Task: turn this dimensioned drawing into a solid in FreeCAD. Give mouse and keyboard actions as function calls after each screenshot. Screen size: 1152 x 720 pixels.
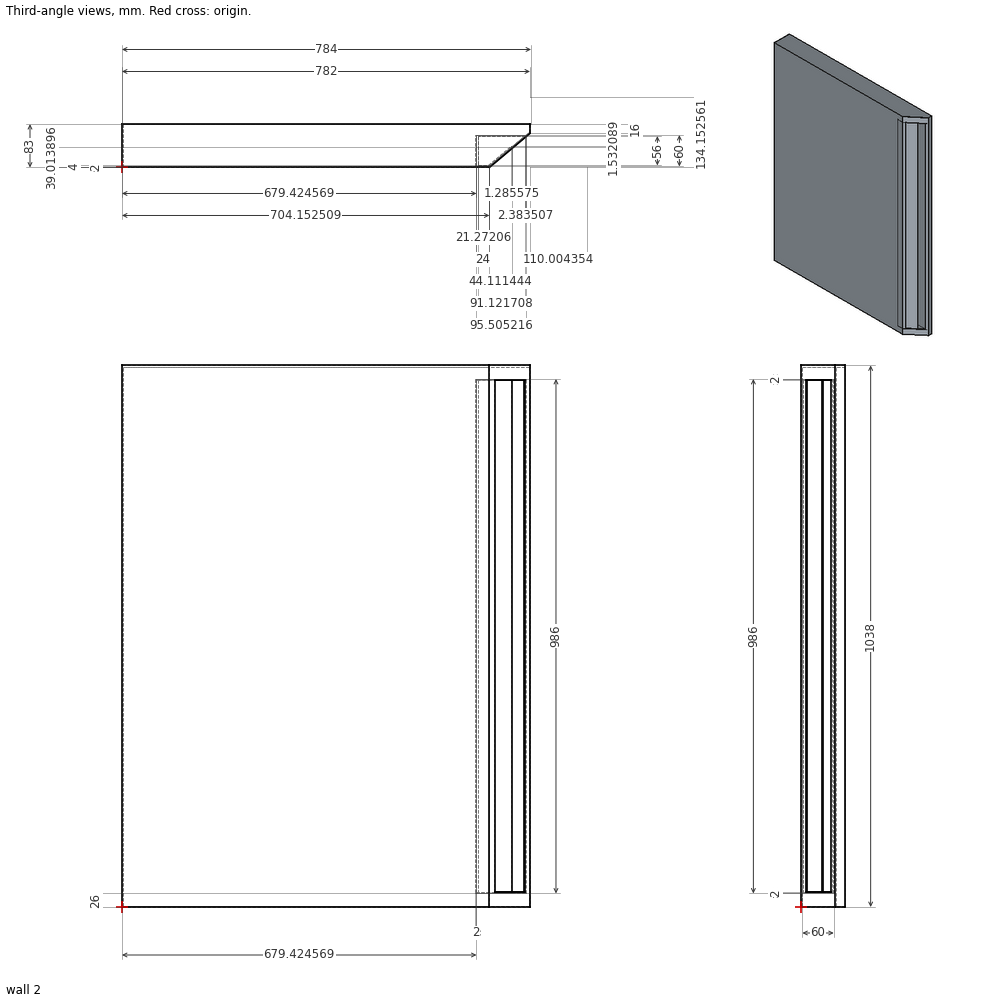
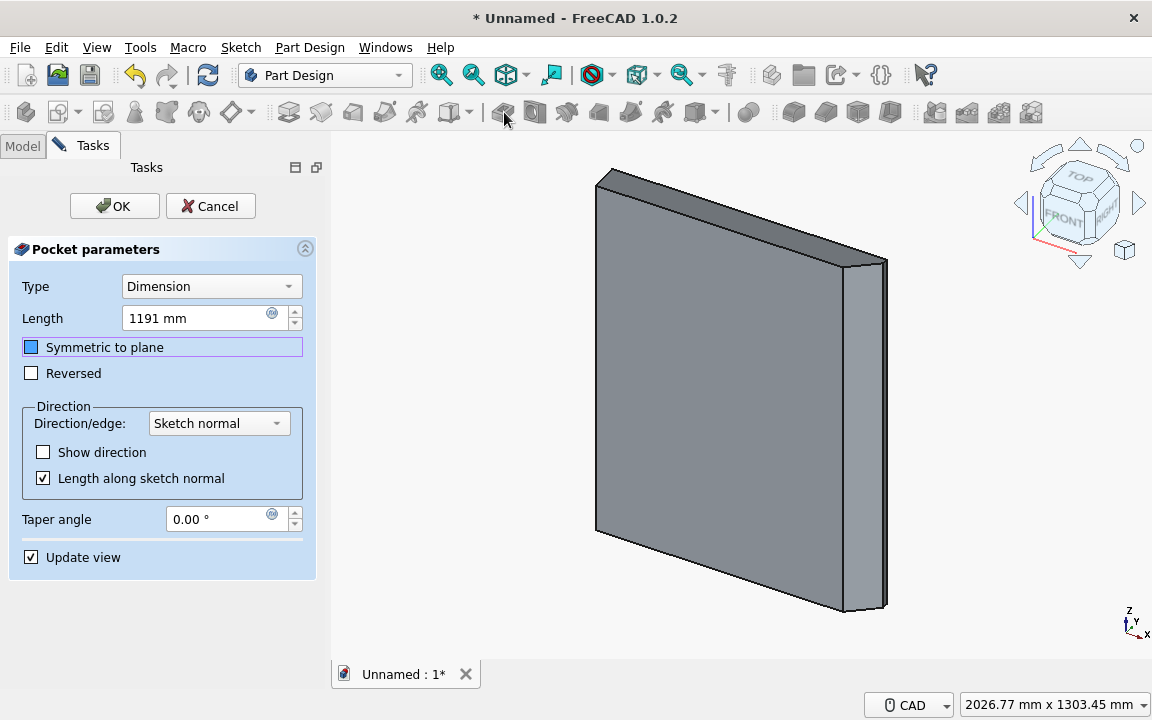
click(115, 206)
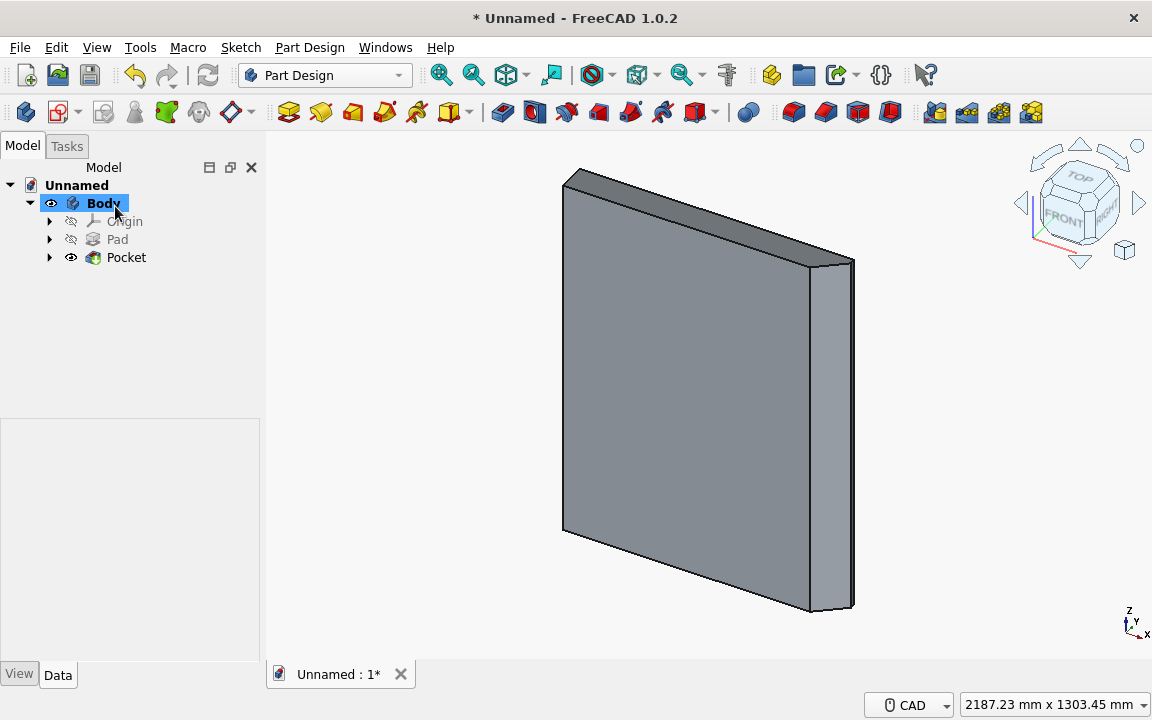
key(0)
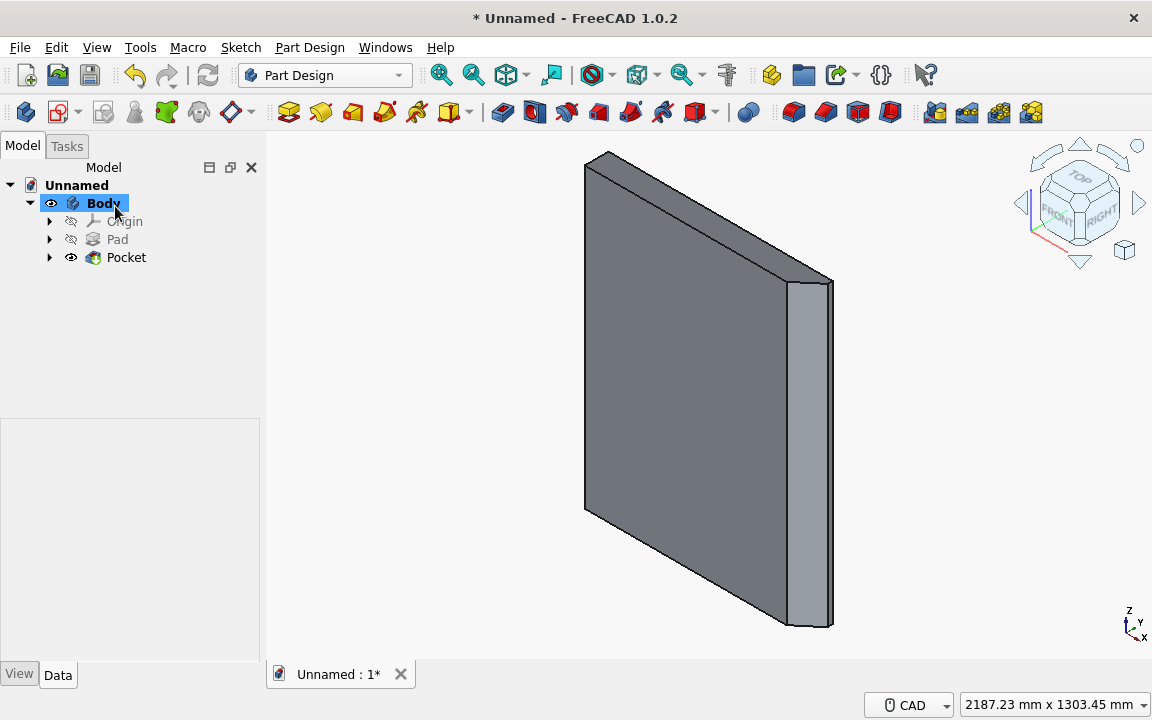
key(2)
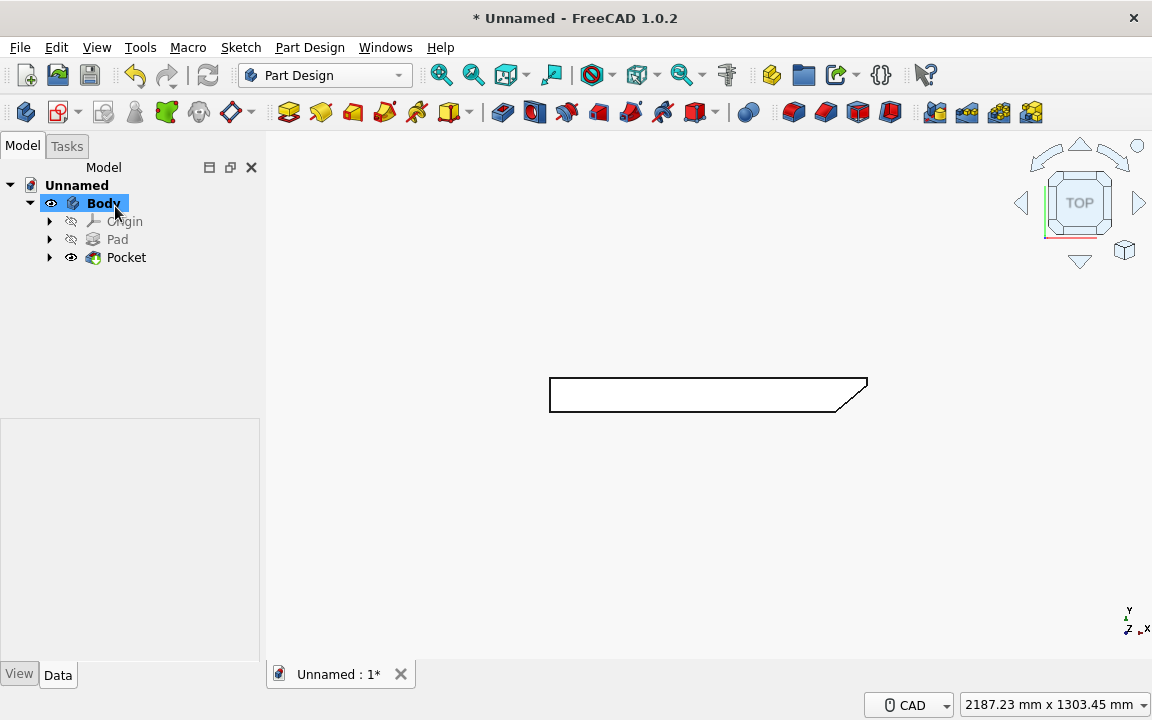
click(442, 76)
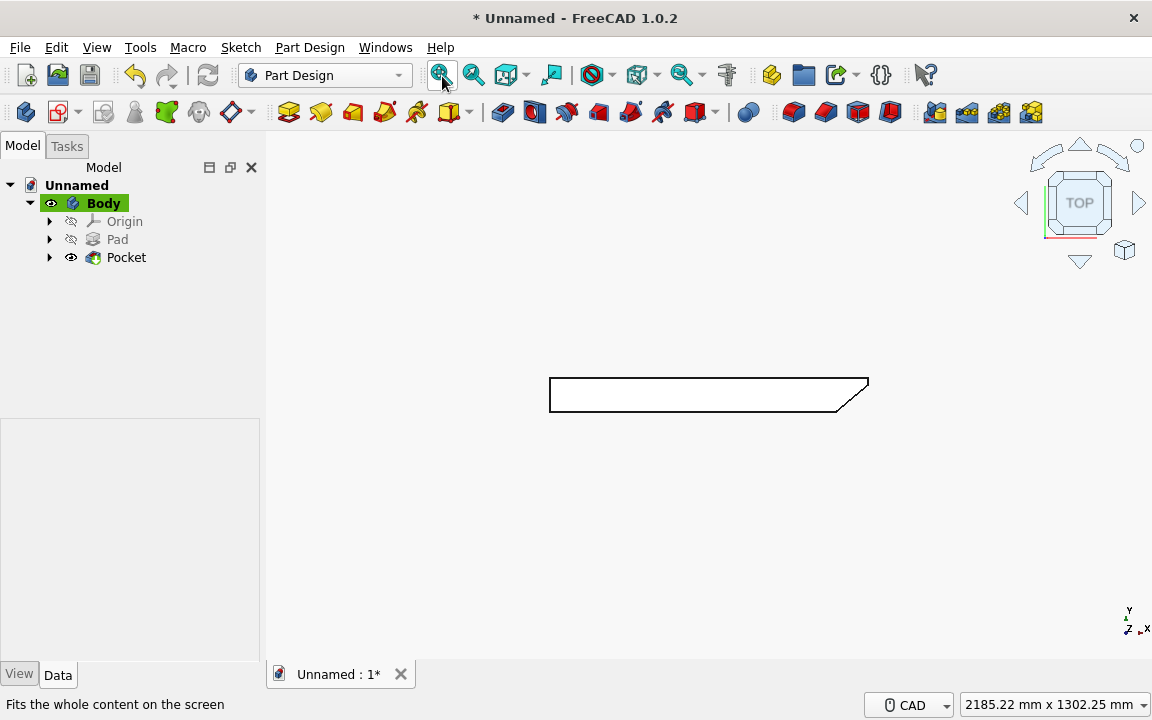
key(1)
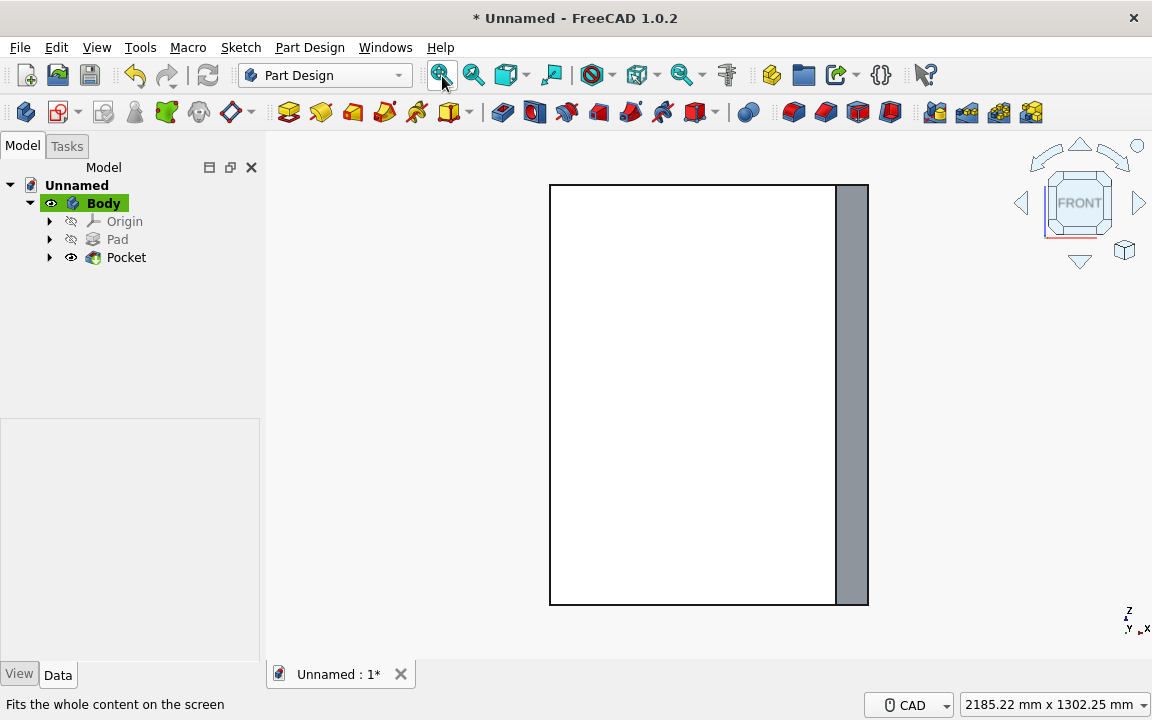
key(3)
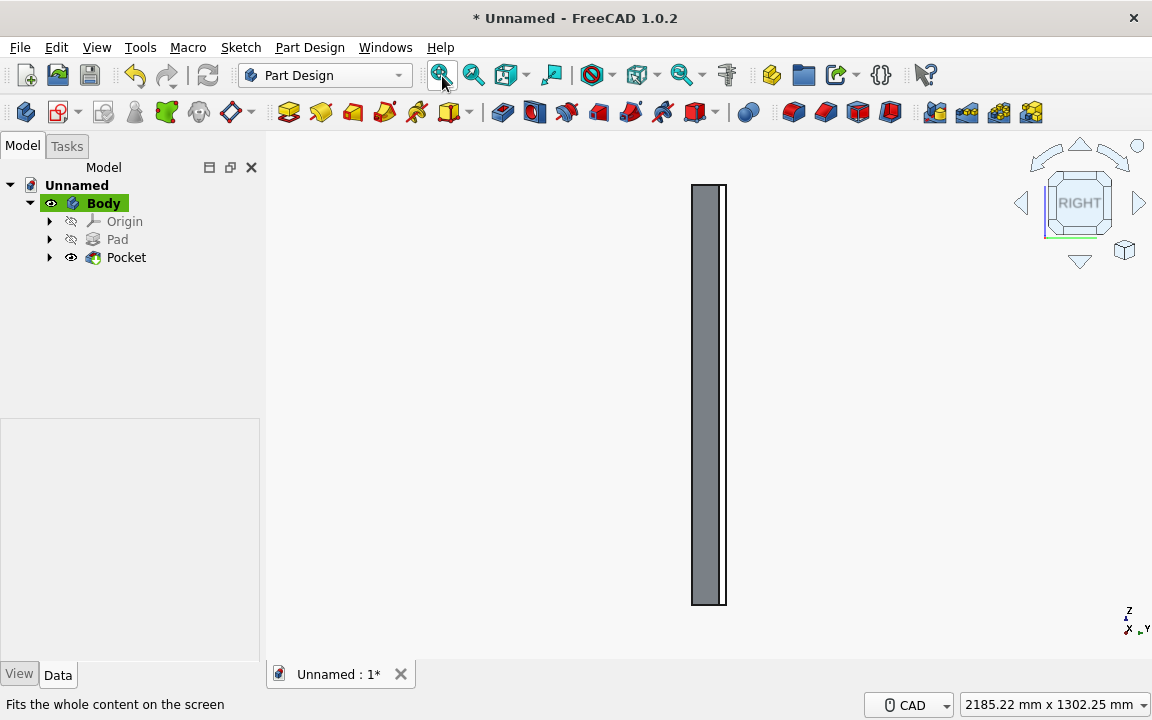
key(5)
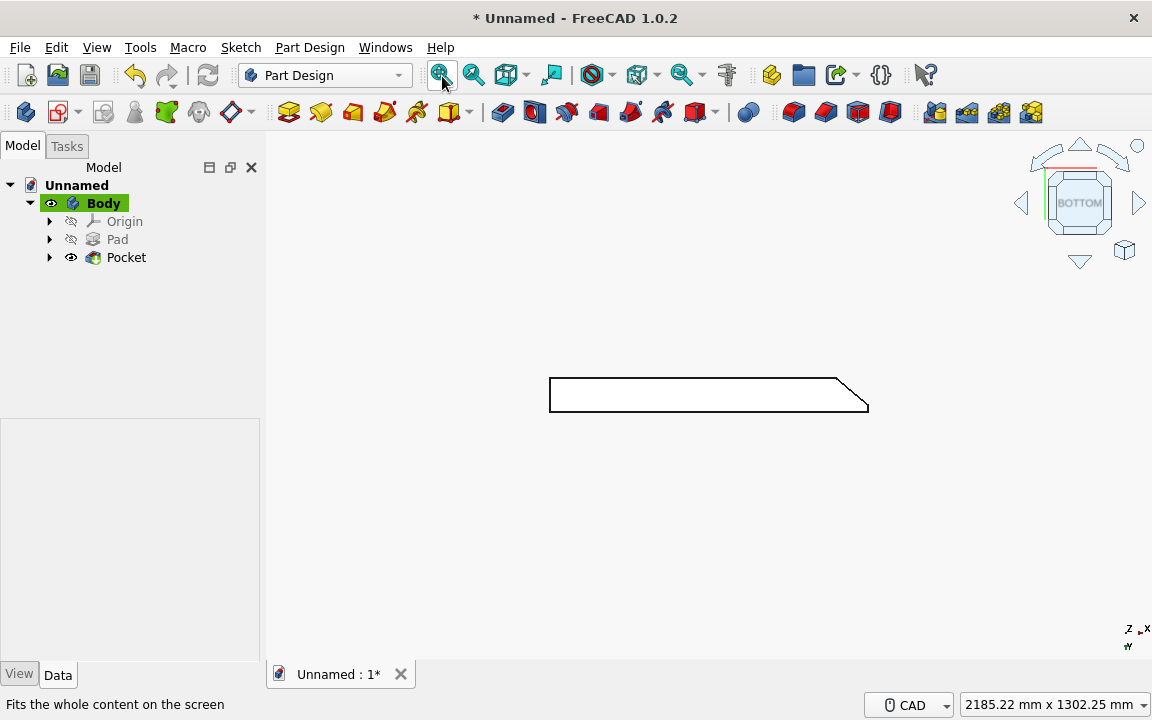
key(v)
key(f)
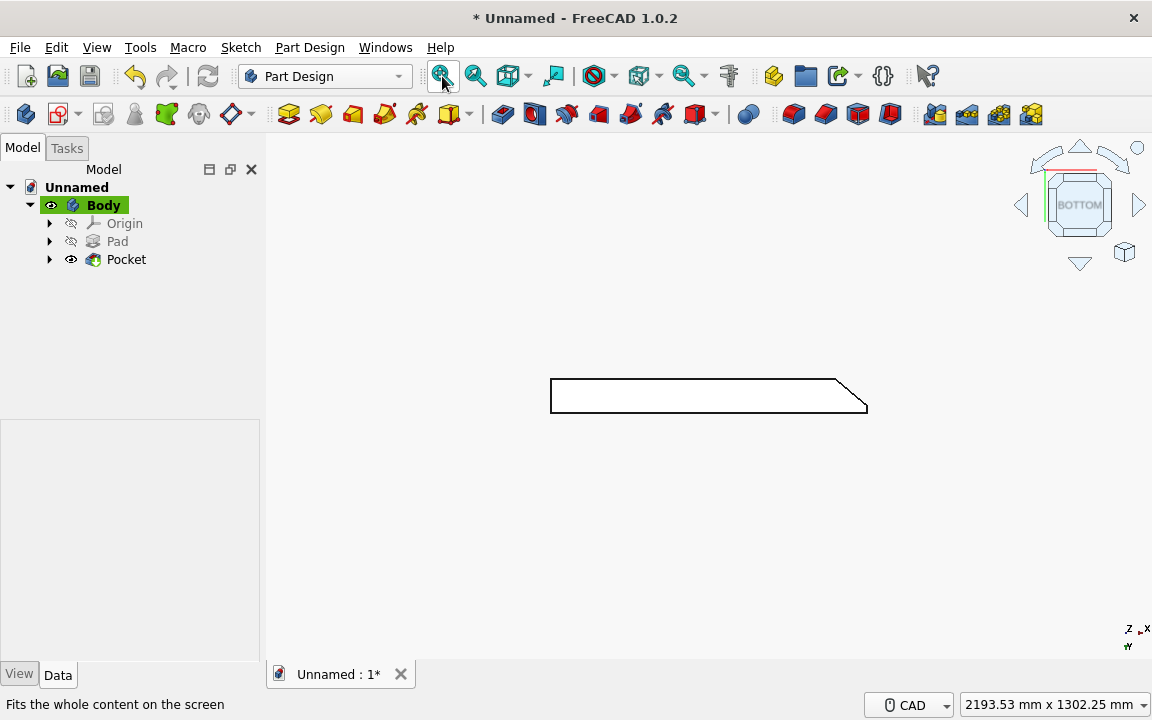
key(4)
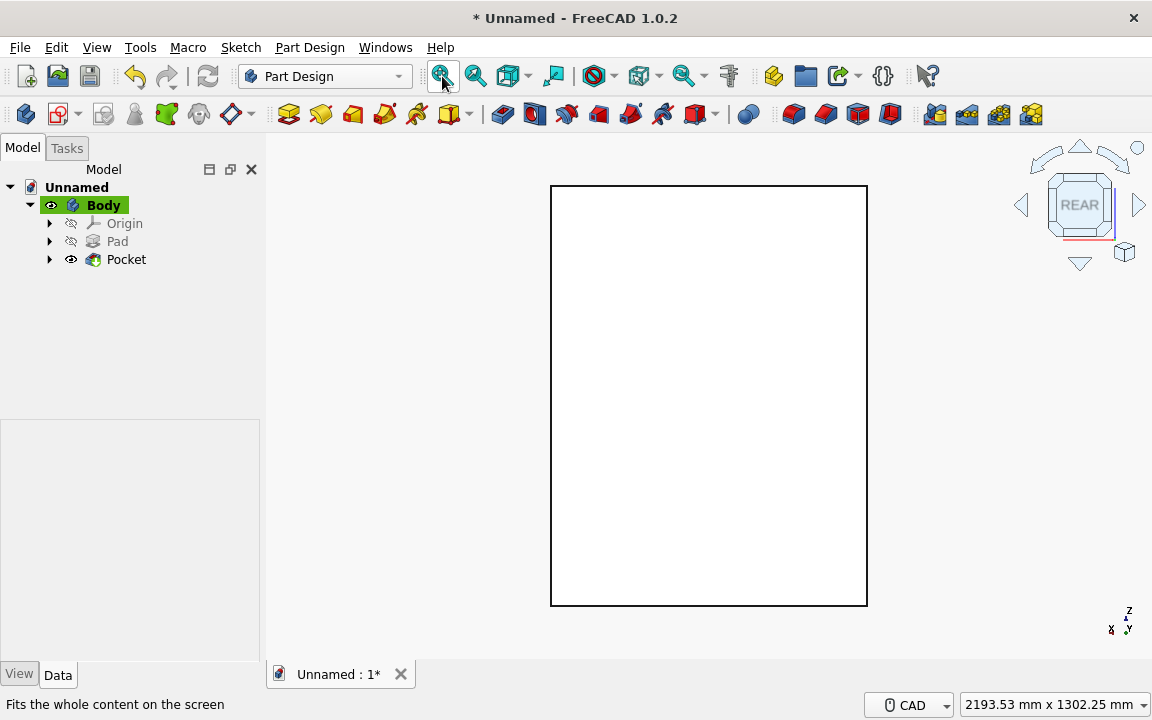
click(709, 395)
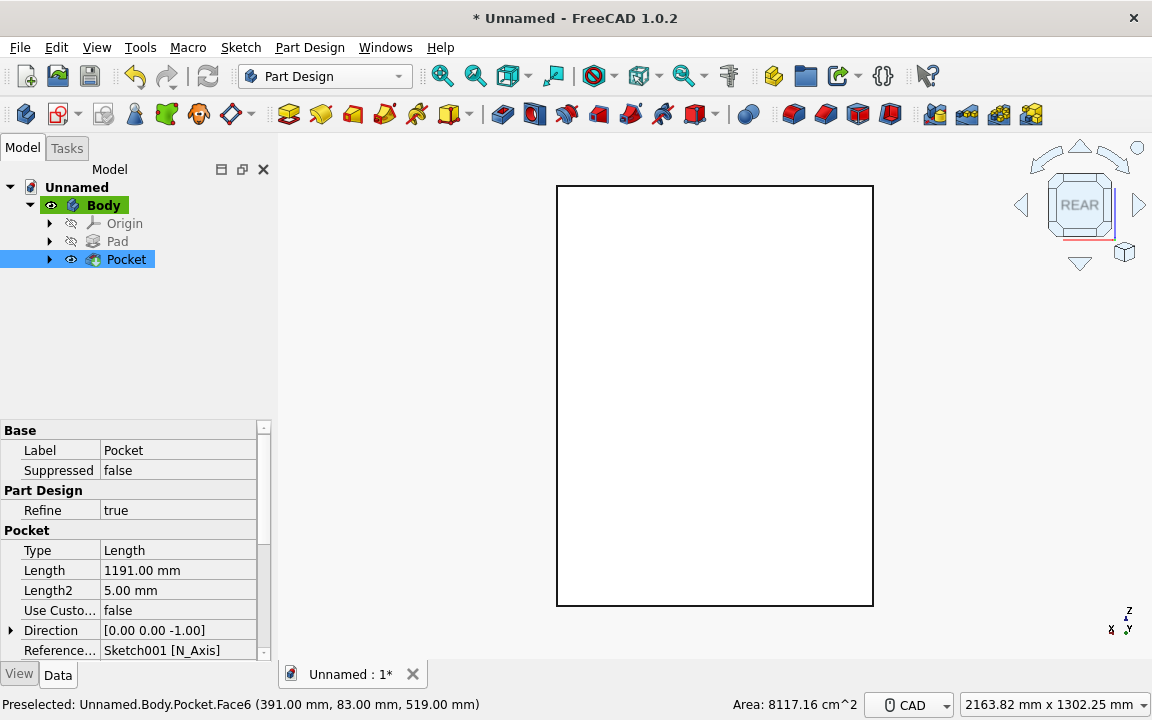
click(890, 114)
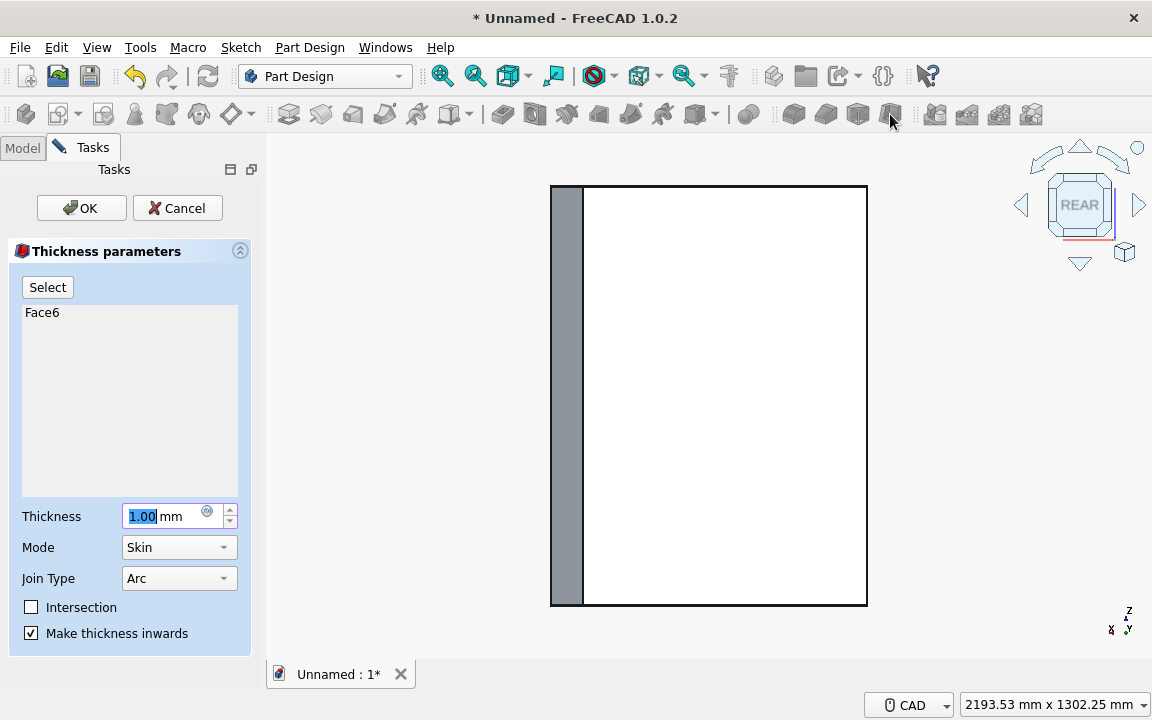
text(2)
key(Tab)